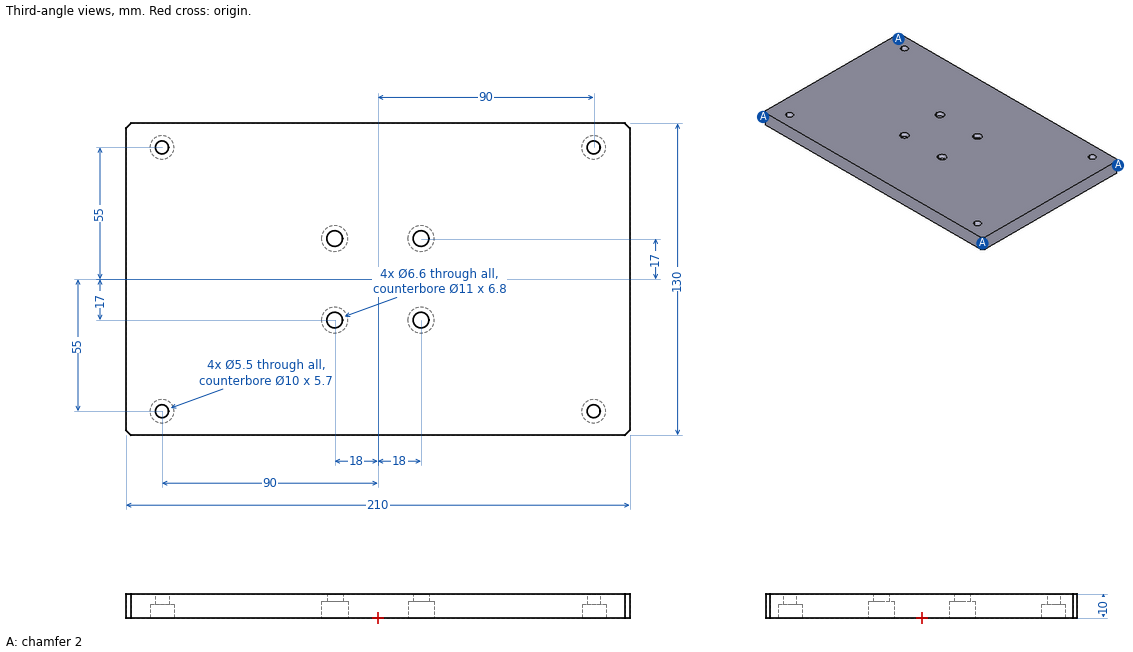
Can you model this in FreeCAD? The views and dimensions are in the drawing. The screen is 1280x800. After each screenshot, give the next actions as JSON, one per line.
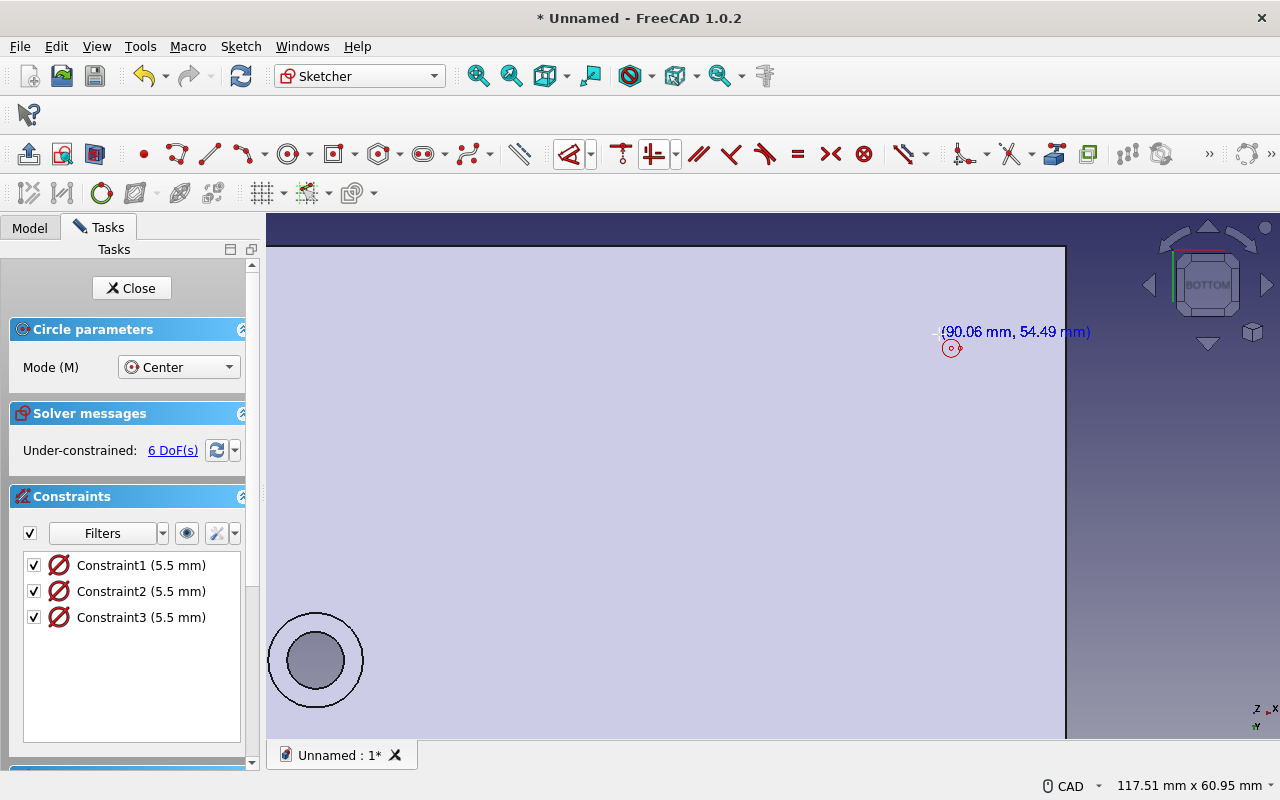
{"action": "scroll", "coordinate": [939, 333], "scroll_direction": "down", "scroll_amount": 6}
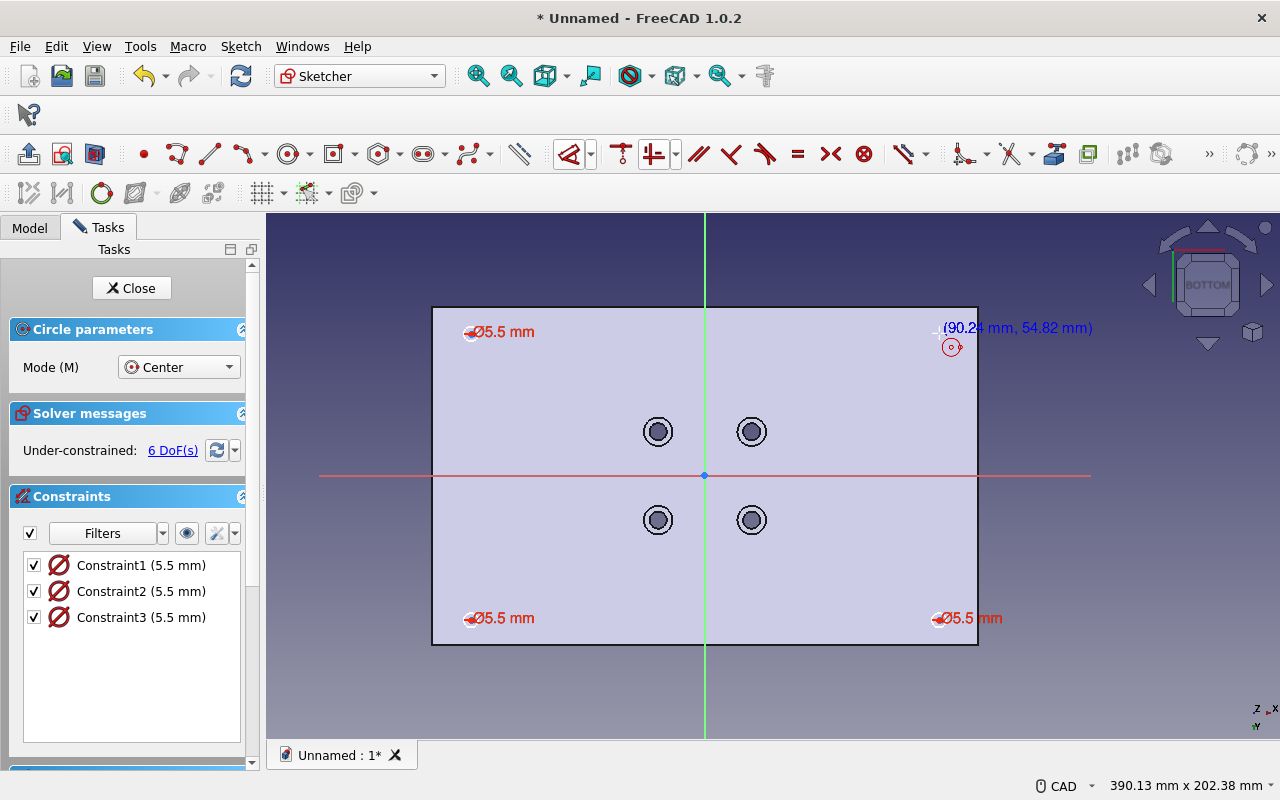
{"action": "left_click", "coordinate": [939, 333]}
{"action": "mouse_move", "coordinate": [944, 328]}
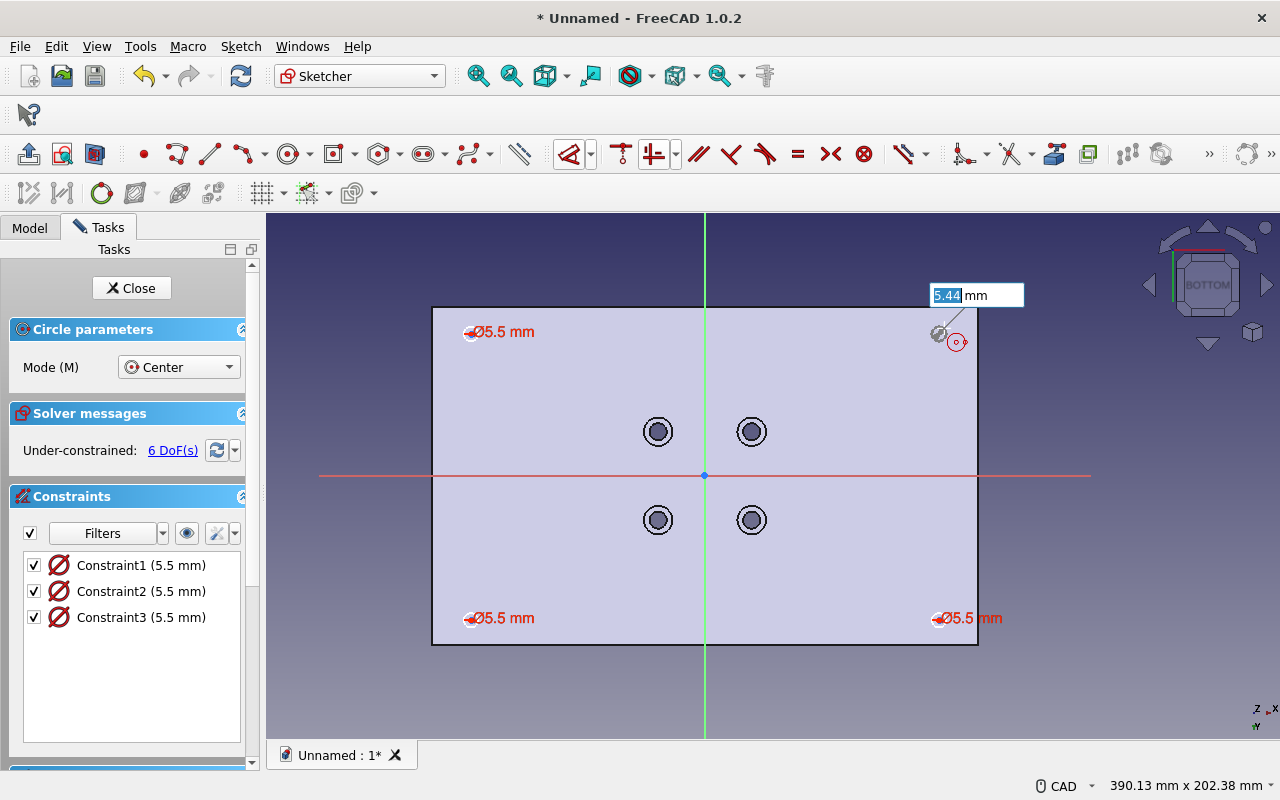
{"action": "type", "text": "5.5"}
{"action": "key", "text": "Return"}
{"action": "key", "text": "Escape"}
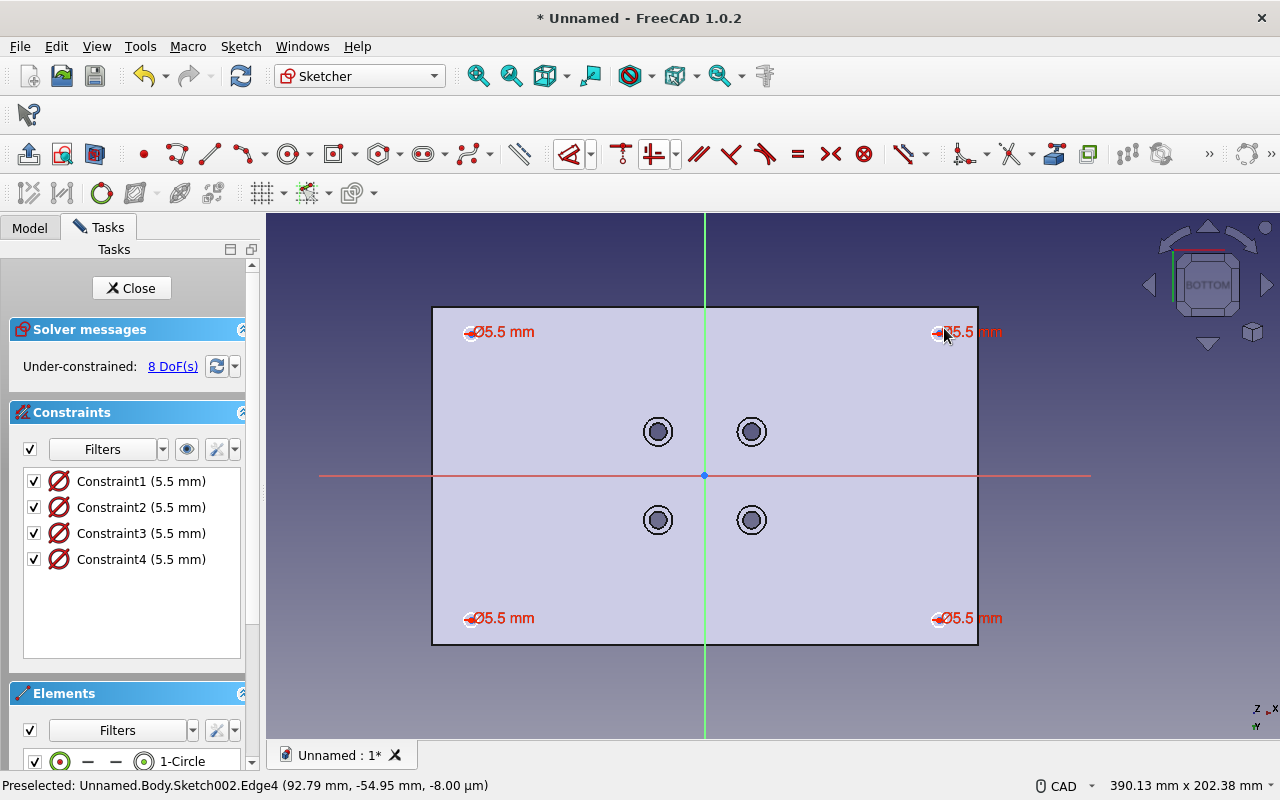
{"action": "left_click", "coordinate": [471, 334]}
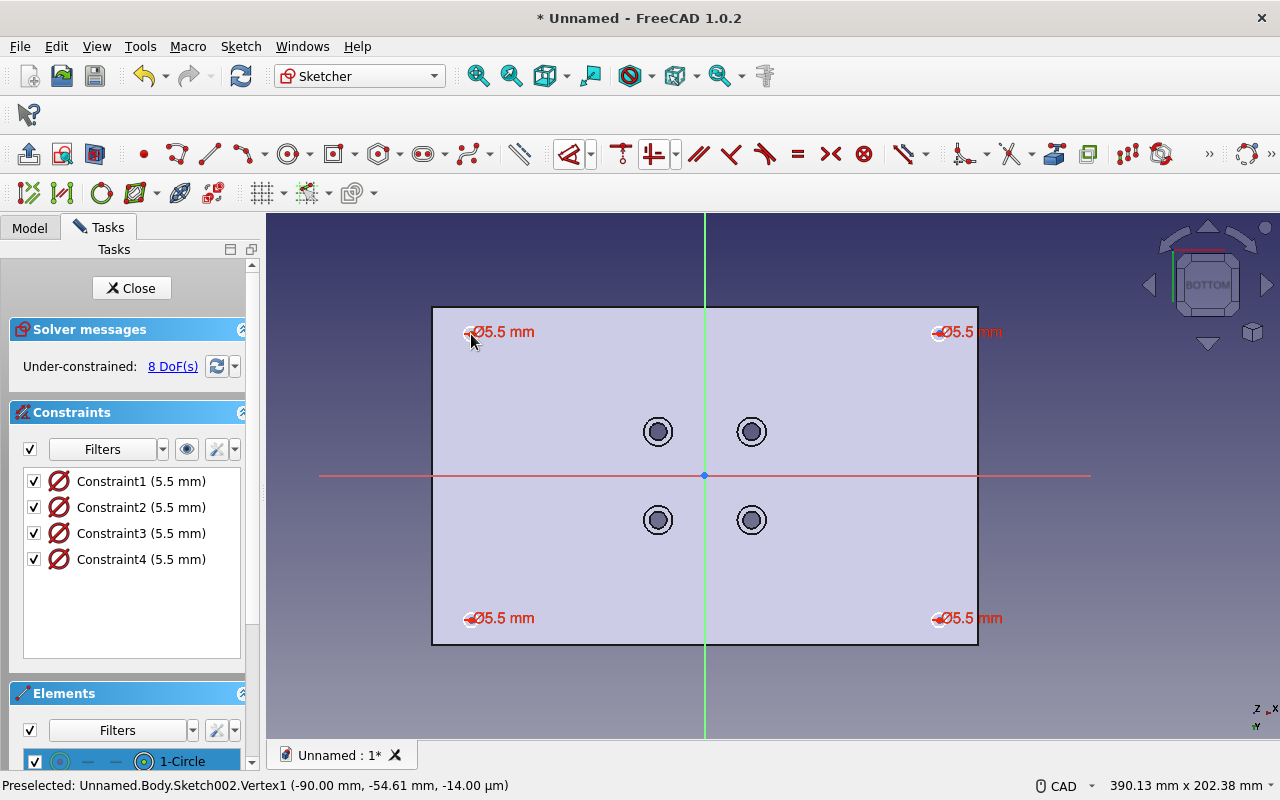
{"action": "left_click", "coordinate": [471, 620]}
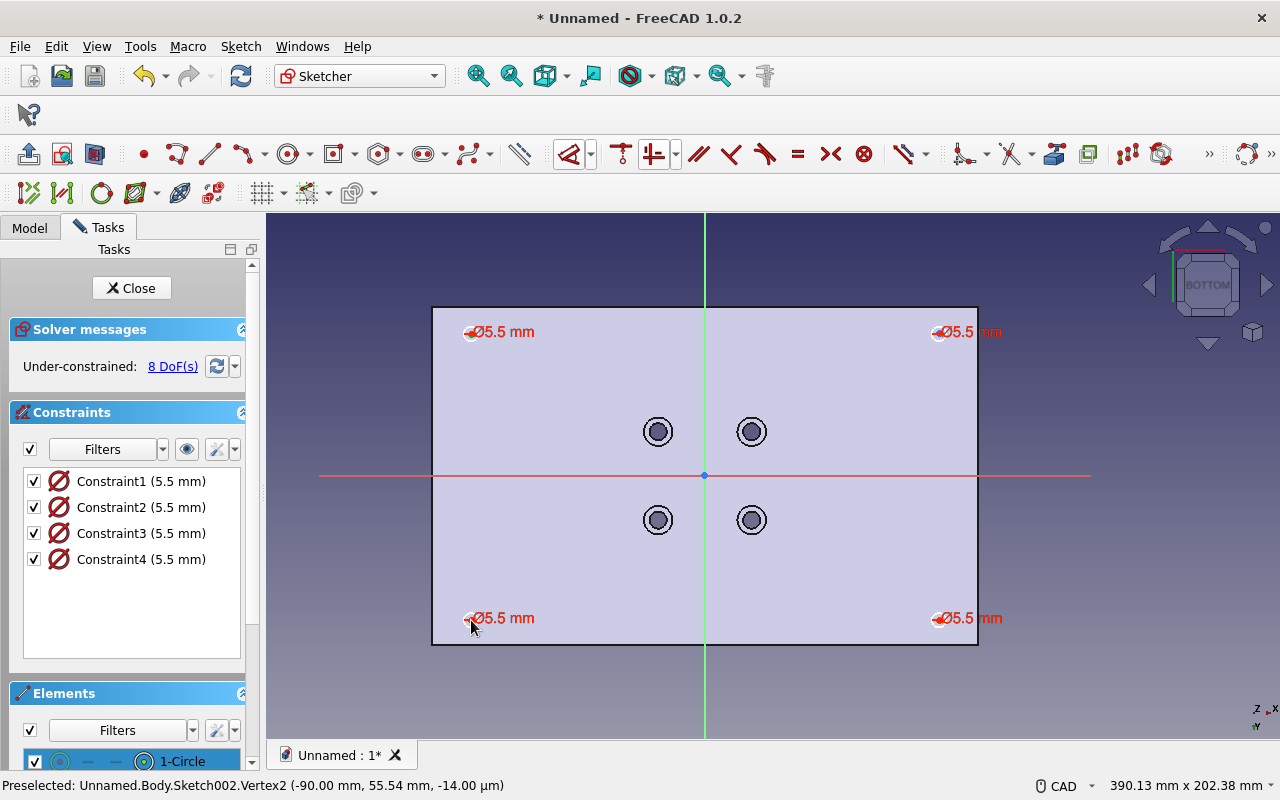
{"action": "key", "text": "v"}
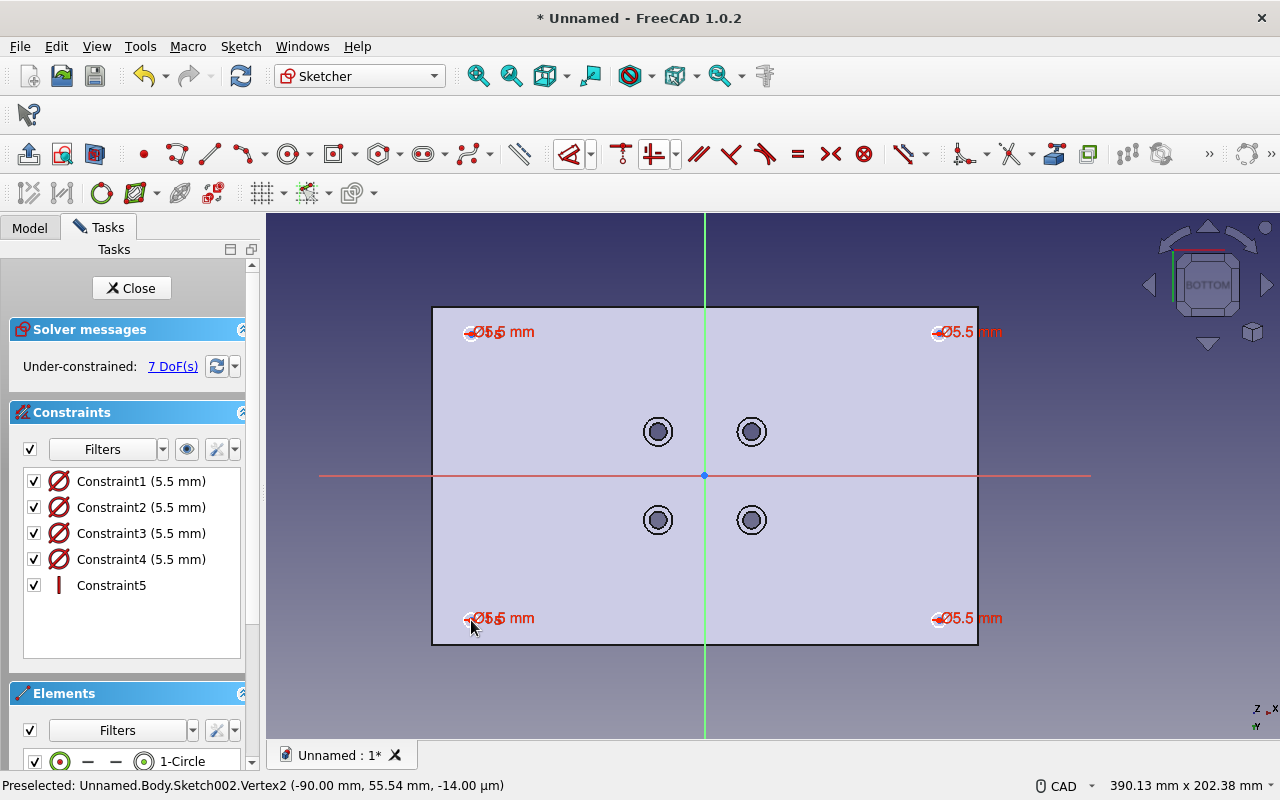
{"action": "left_click", "coordinate": [471, 620]}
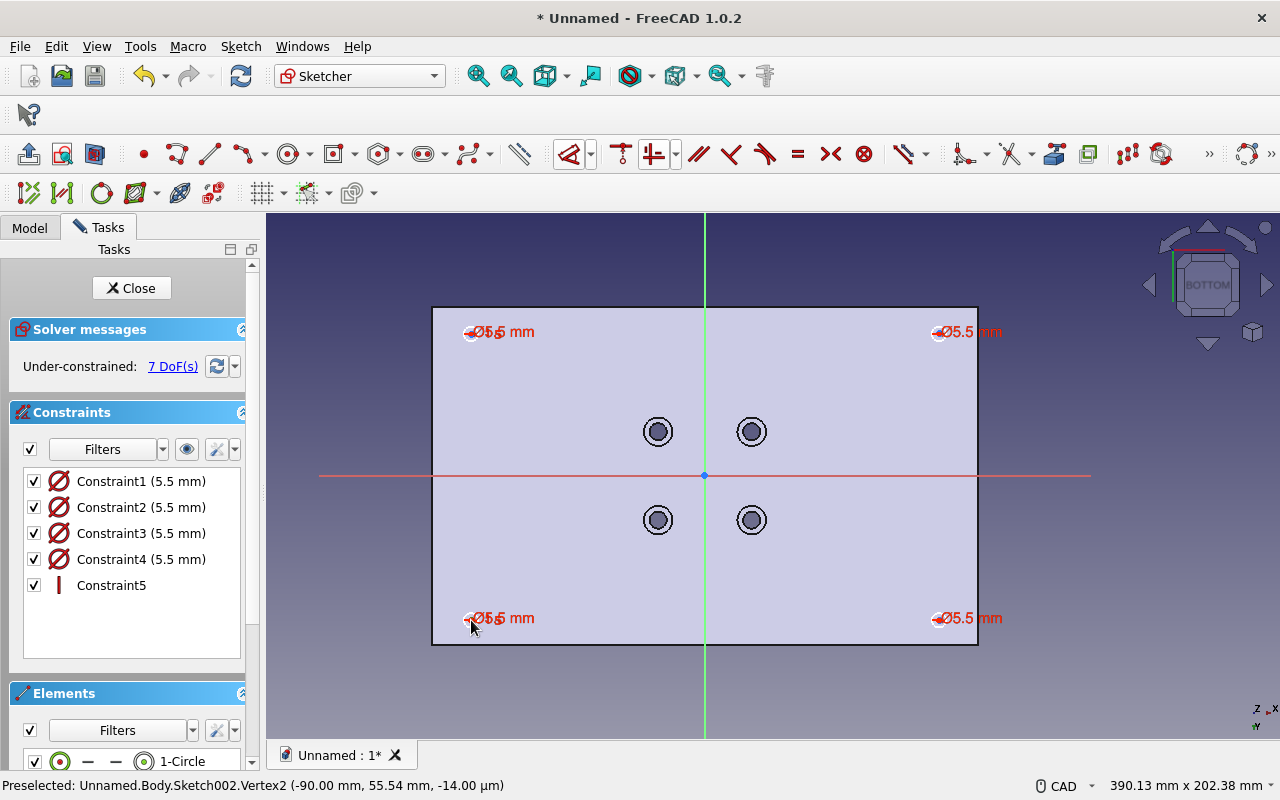
{"action": "left_click", "coordinate": [939, 620]}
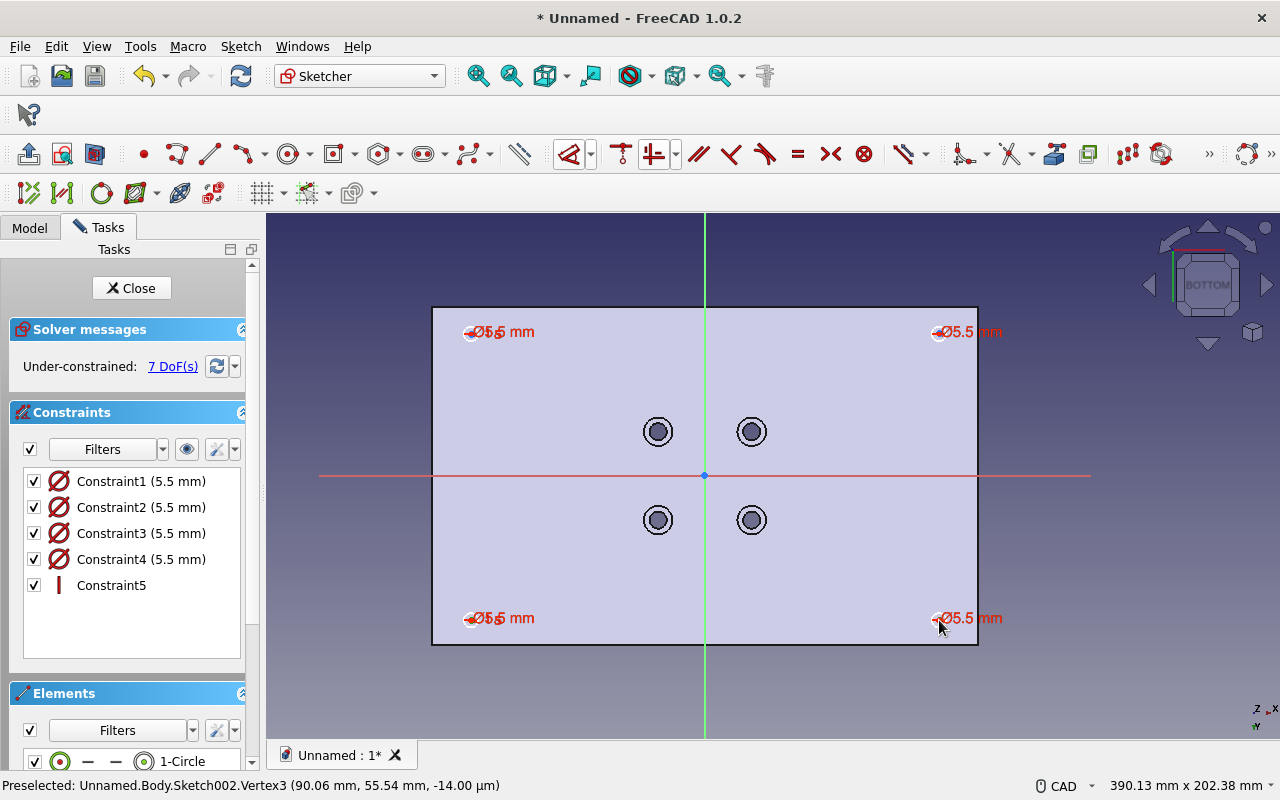
{"action": "key", "text": "h"}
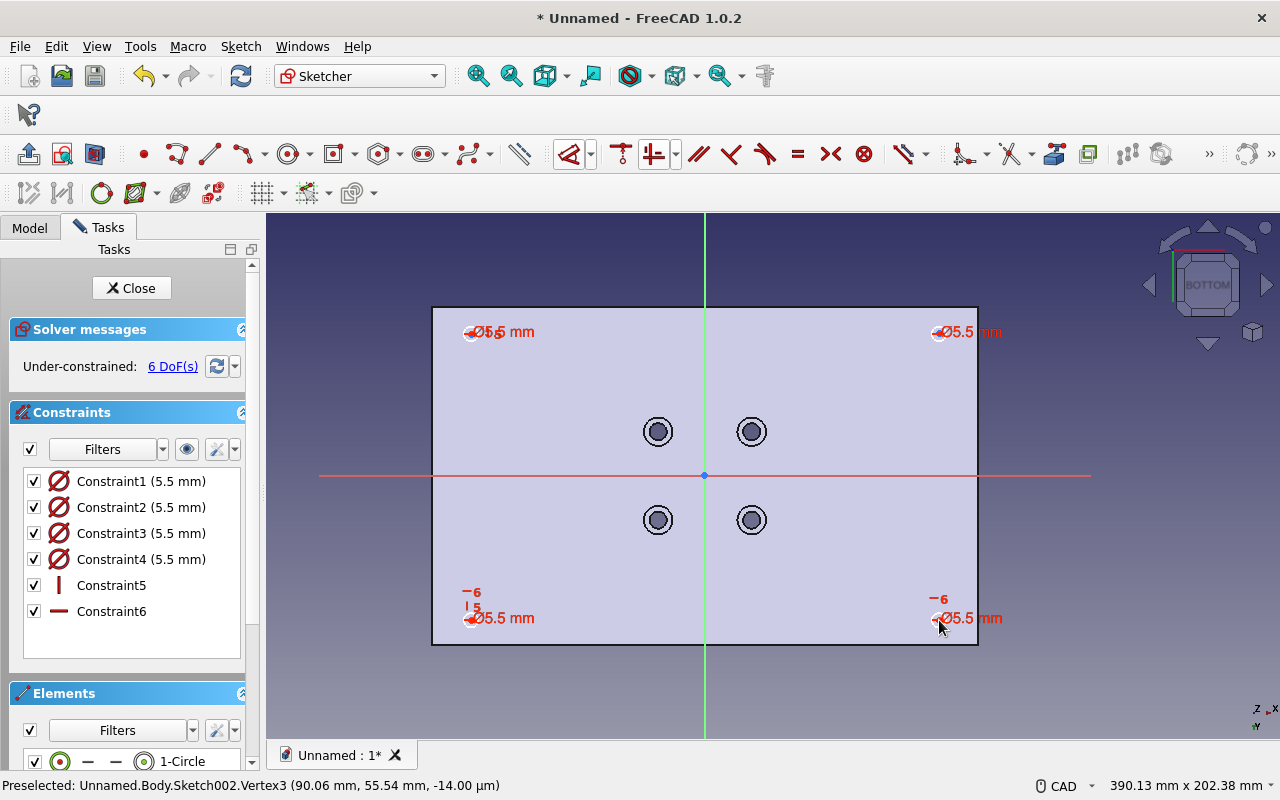
{"action": "left_click", "coordinate": [939, 620]}